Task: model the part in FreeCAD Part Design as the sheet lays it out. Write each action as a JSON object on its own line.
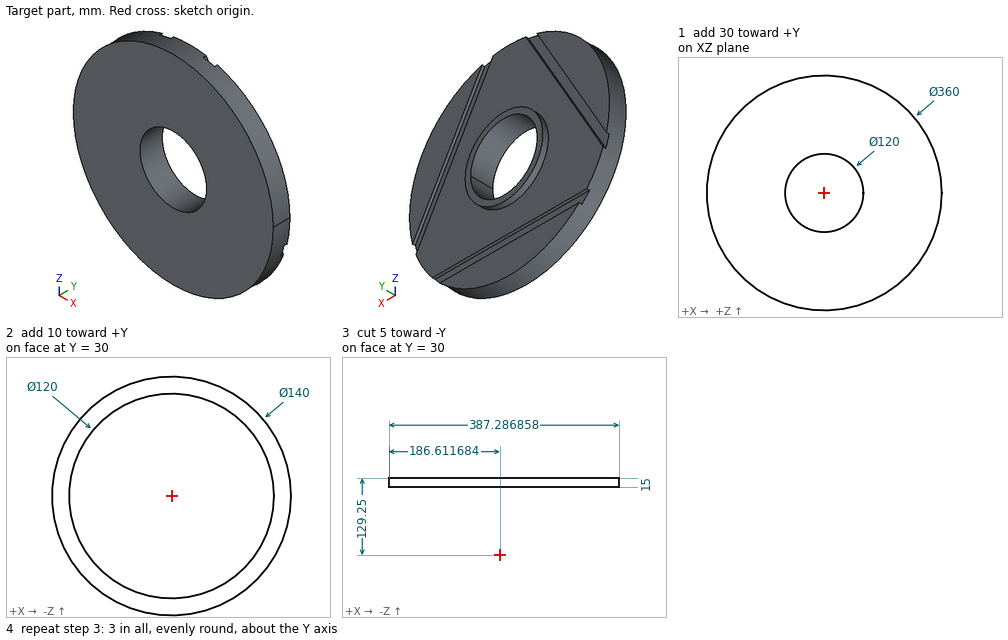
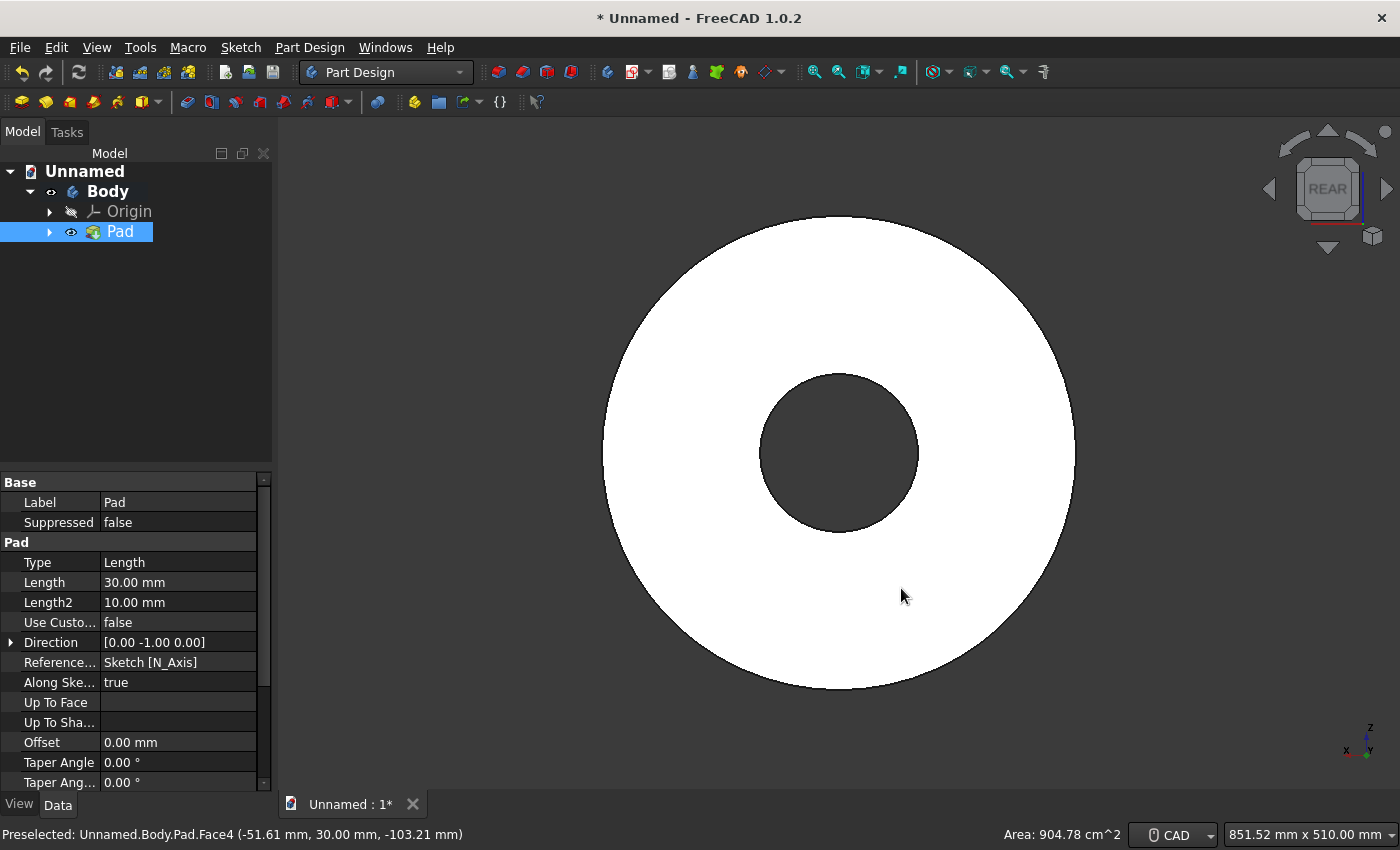
{"action": "left_click", "coordinate": [632, 72]}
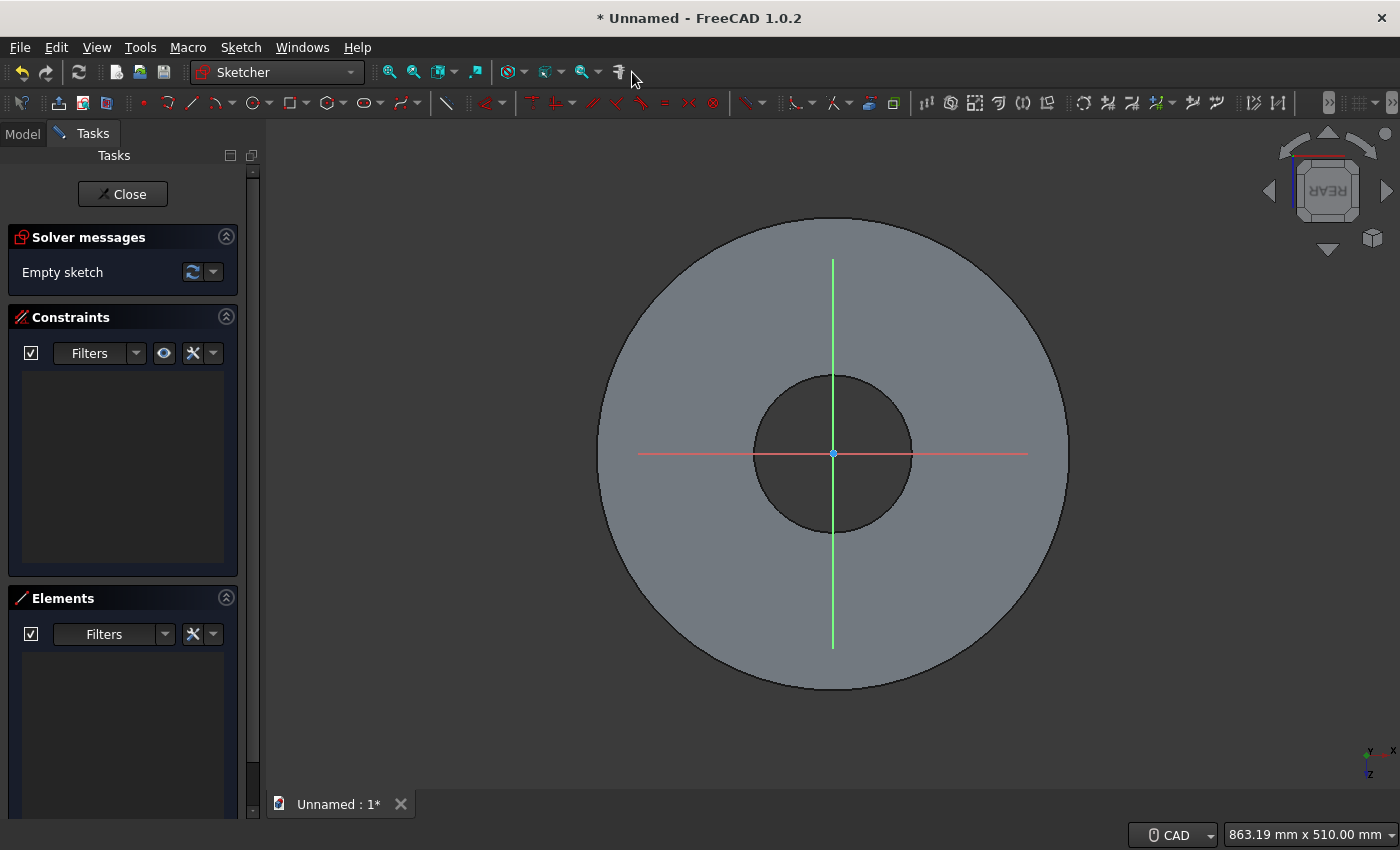
{"action": "scroll", "coordinate": [889, 454], "scroll_direction": "up", "scroll_amount": 4}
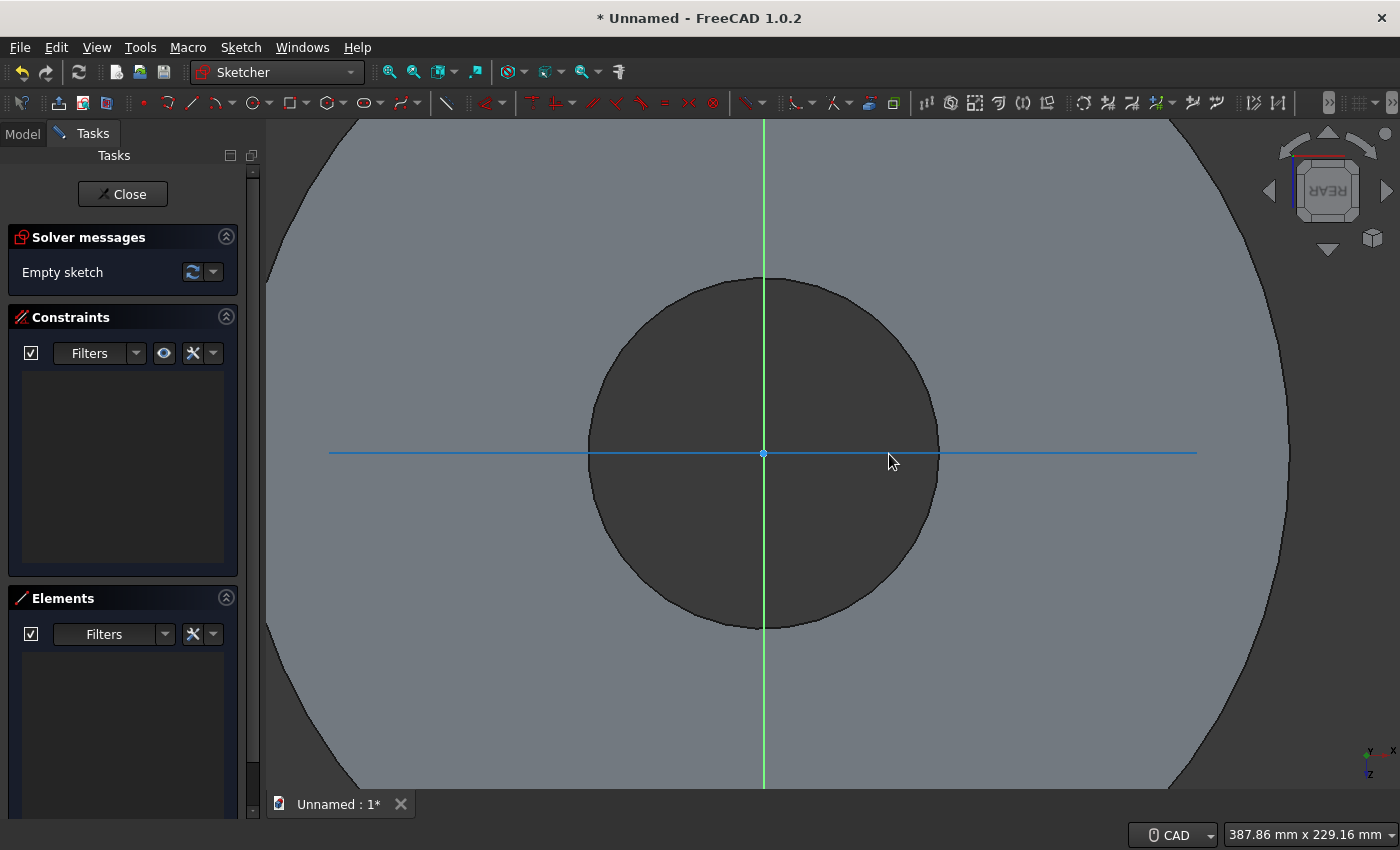
{"action": "left_click", "coordinate": [254, 104]}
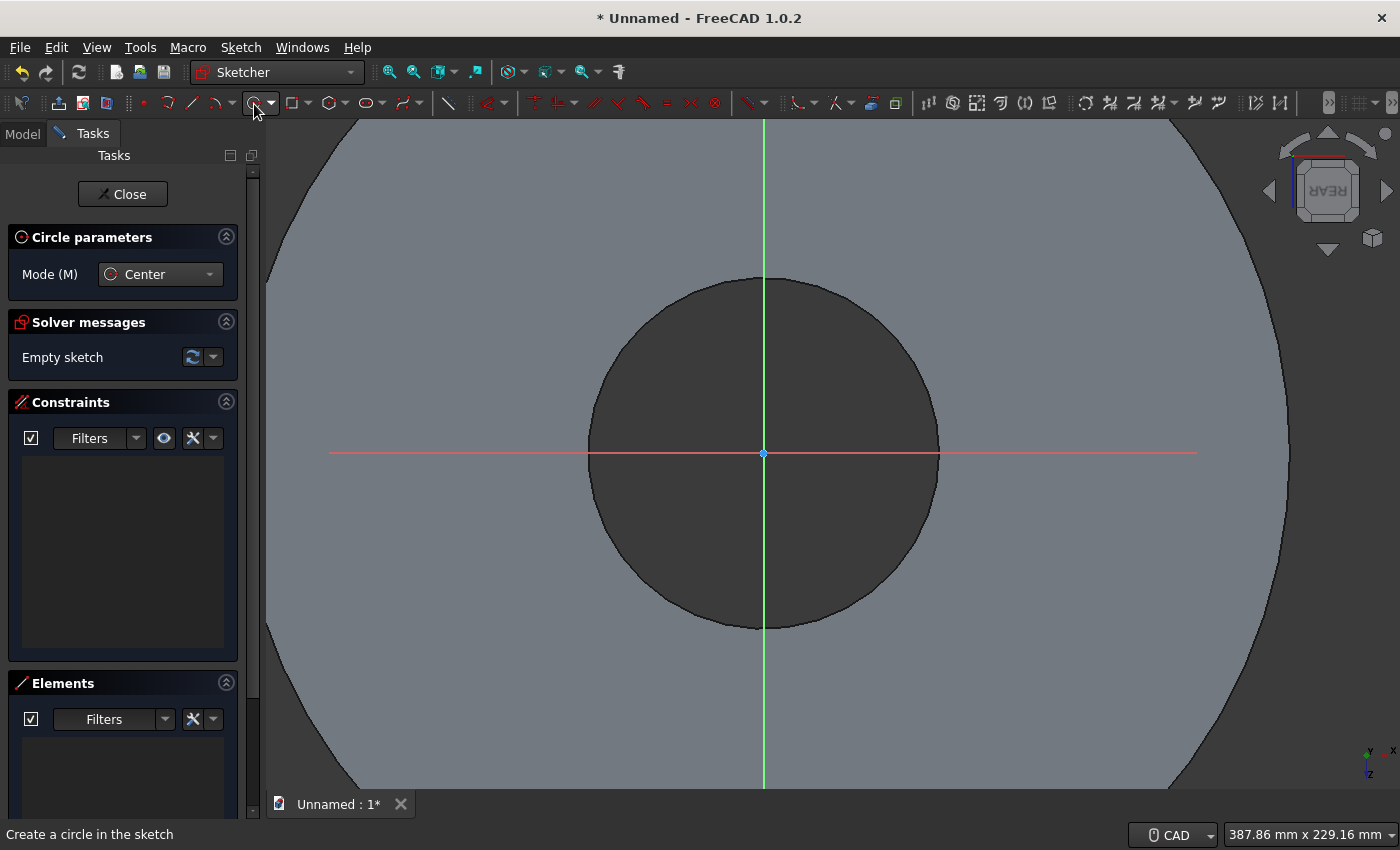
{"action": "left_click", "coordinate": [764, 453]}
{"action": "mouse_move", "coordinate": [908, 309]}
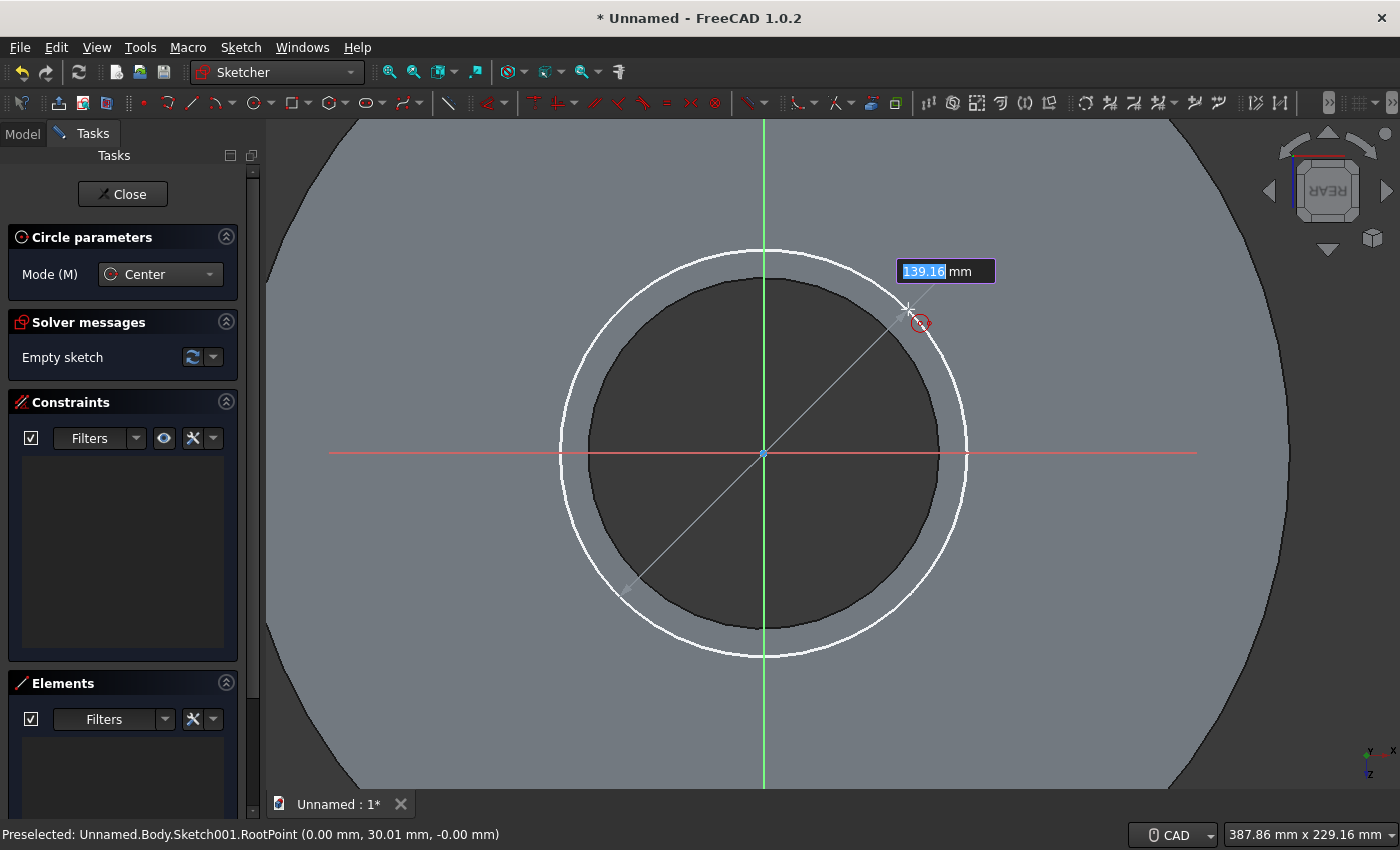
{"action": "type", "text": "140"}
{"action": "key", "text": "Return"}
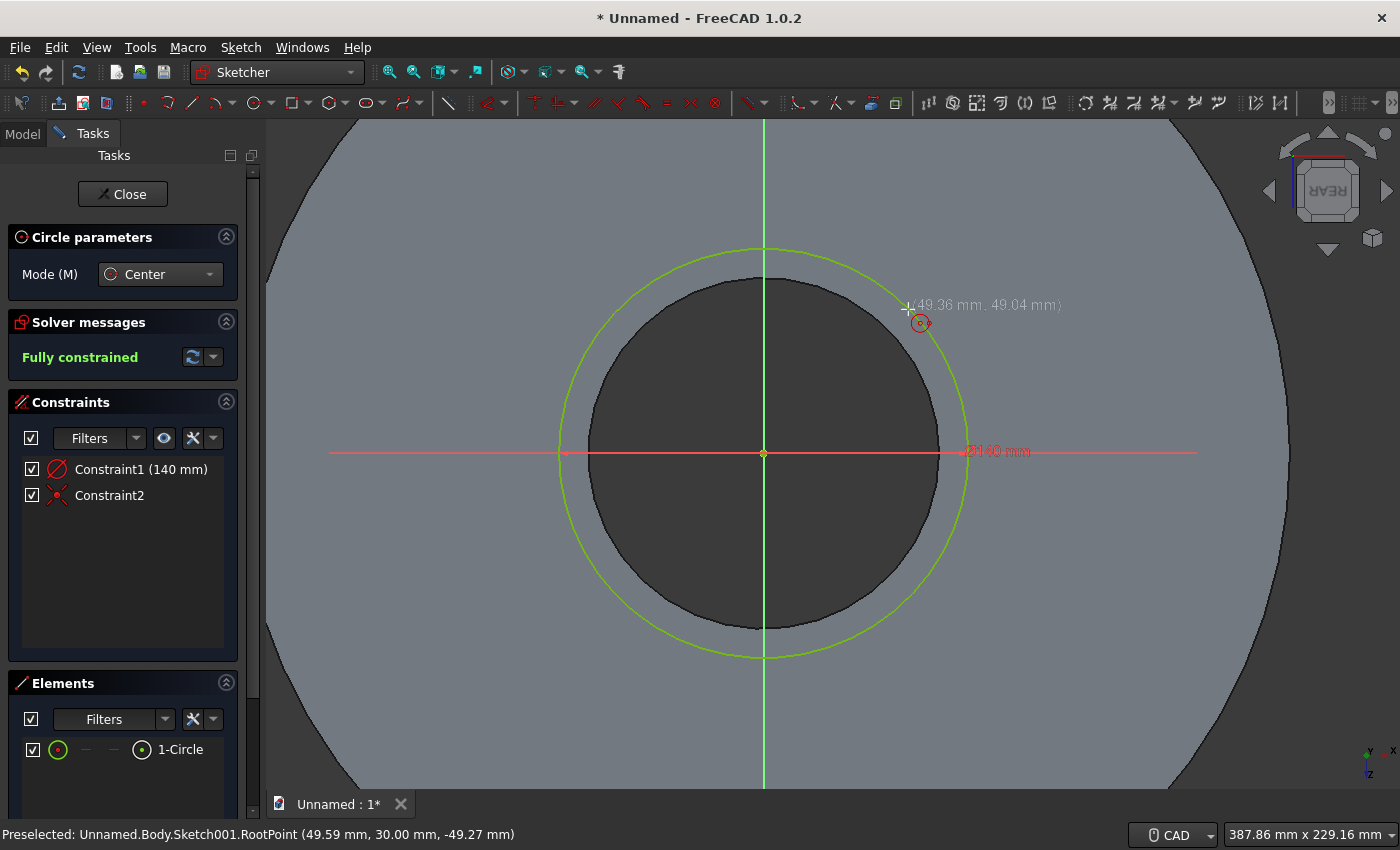
{"action": "left_click", "coordinate": [764, 453]}
{"action": "mouse_move", "coordinate": [888, 329]}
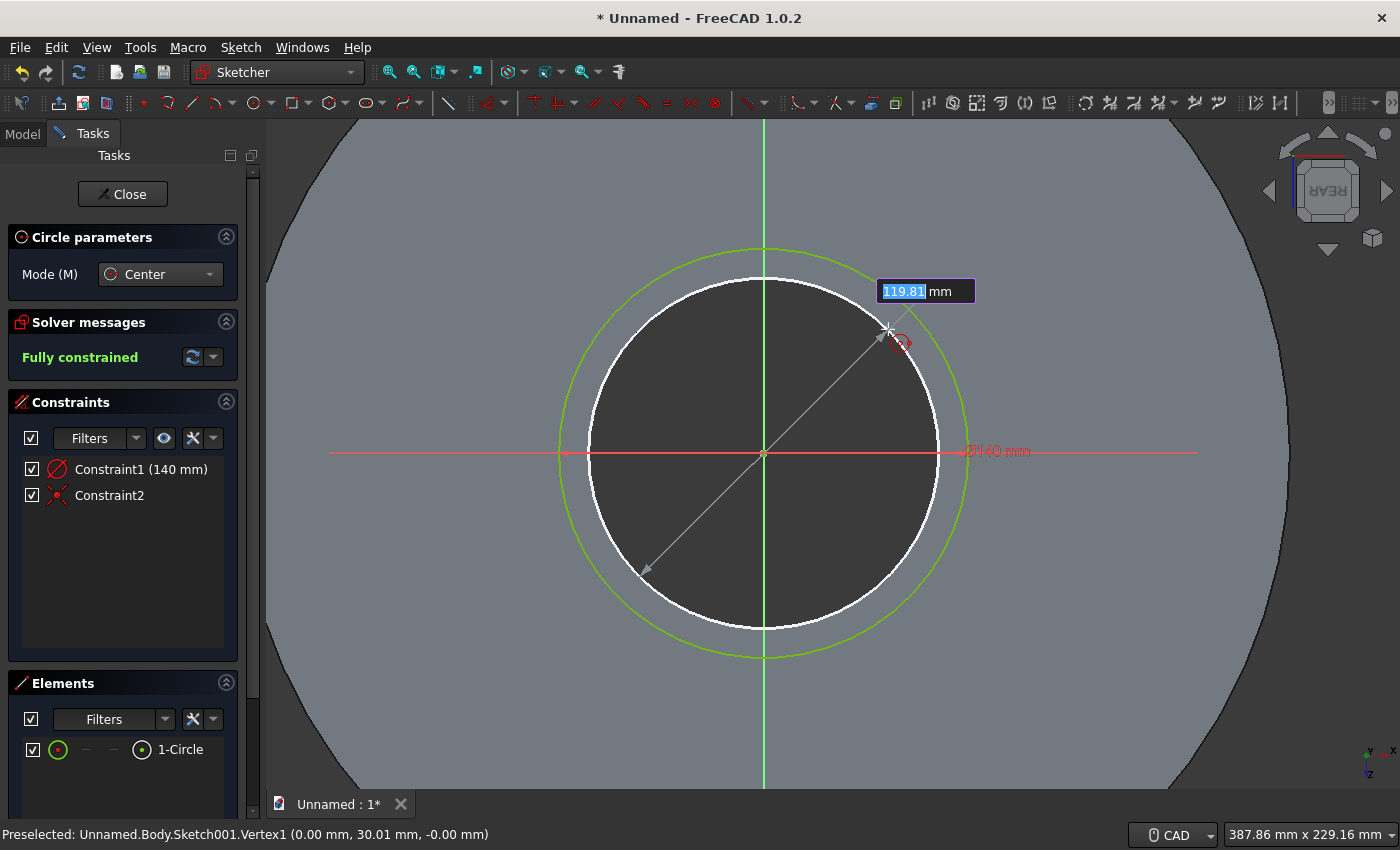
{"action": "type", "text": "120"}
{"action": "key", "text": "Return"}
{"action": "key", "text": "Escape"}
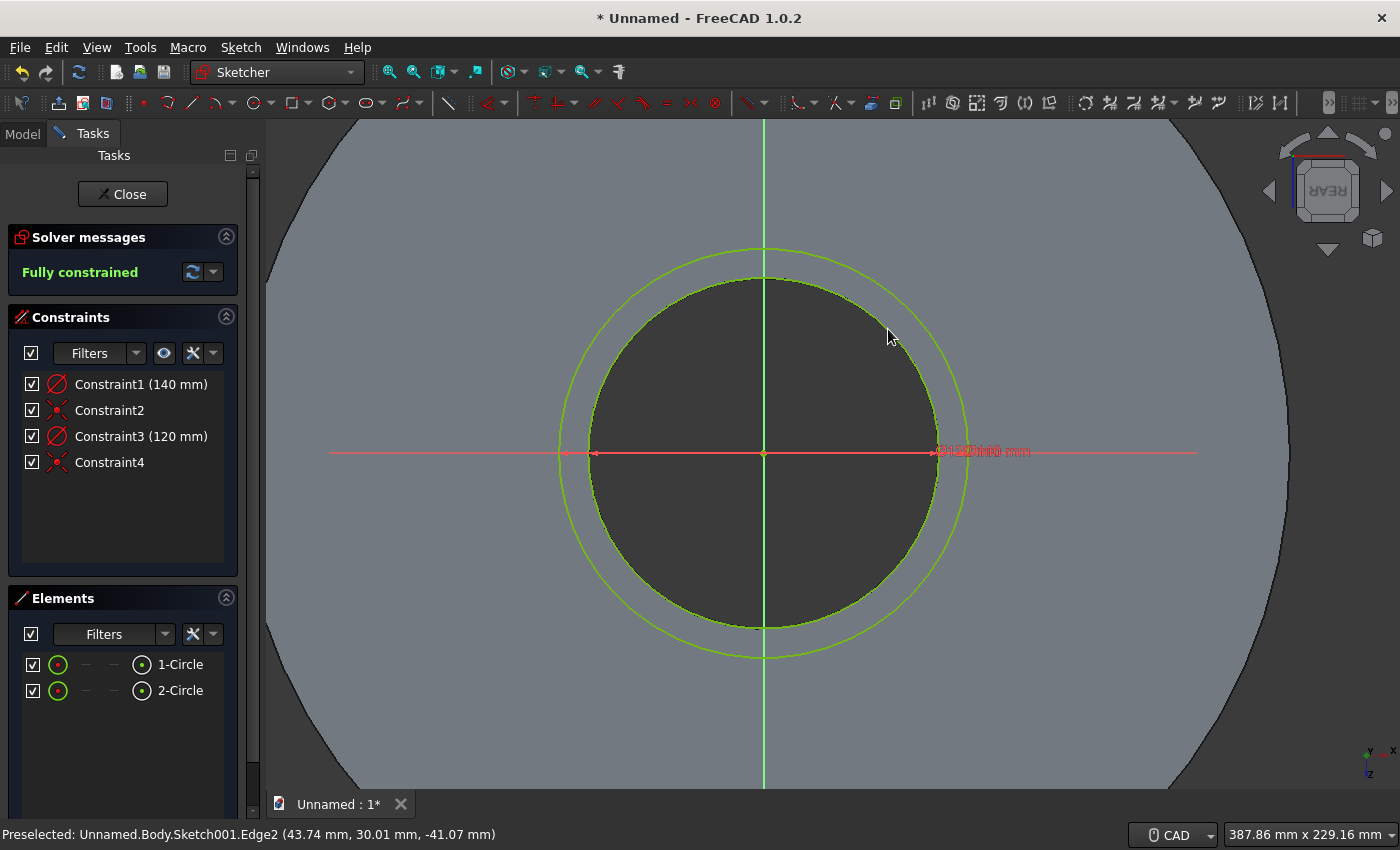
{"action": "left_click", "coordinate": [123, 194]}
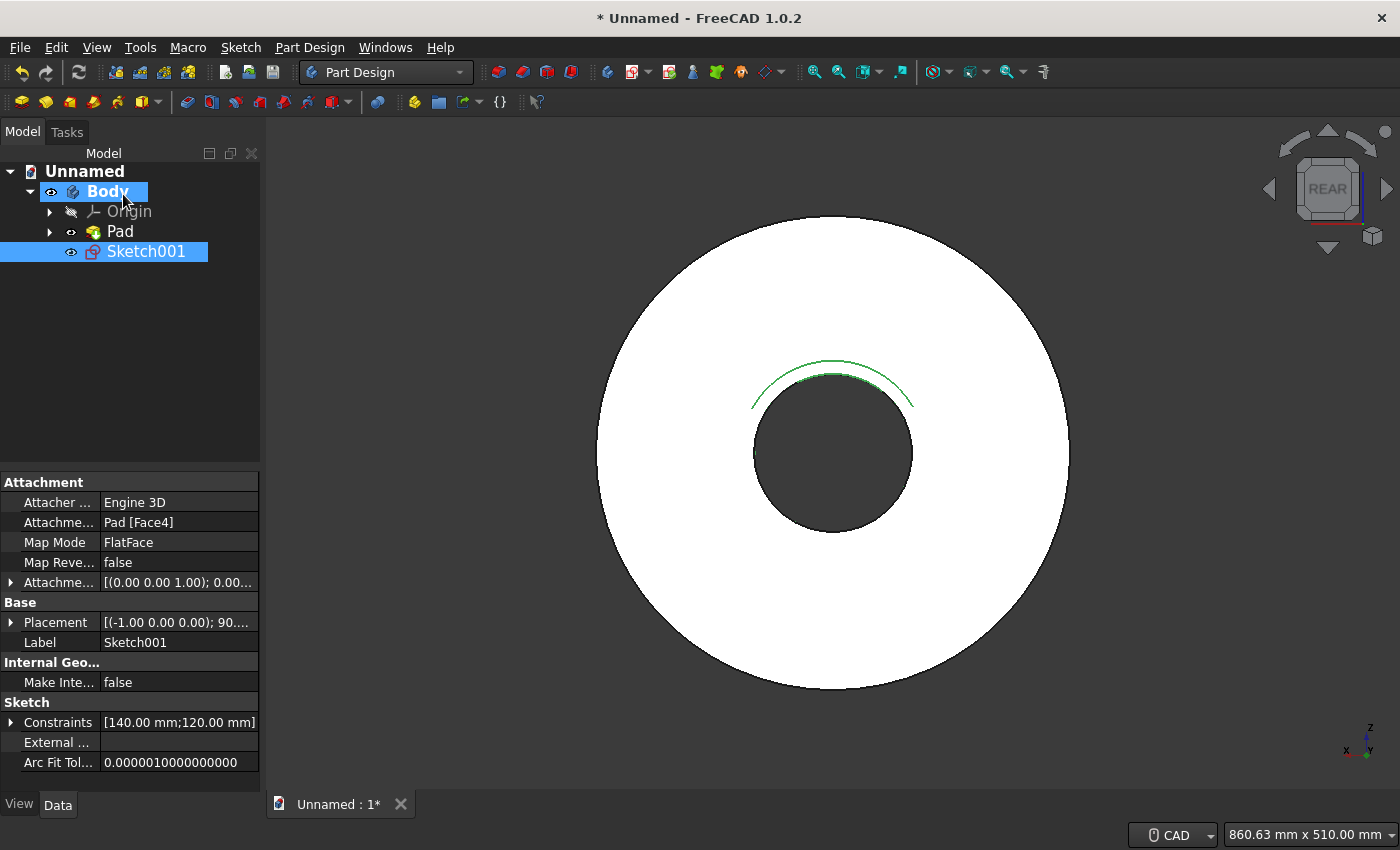
{"action": "left_click", "coordinate": [22, 102]}